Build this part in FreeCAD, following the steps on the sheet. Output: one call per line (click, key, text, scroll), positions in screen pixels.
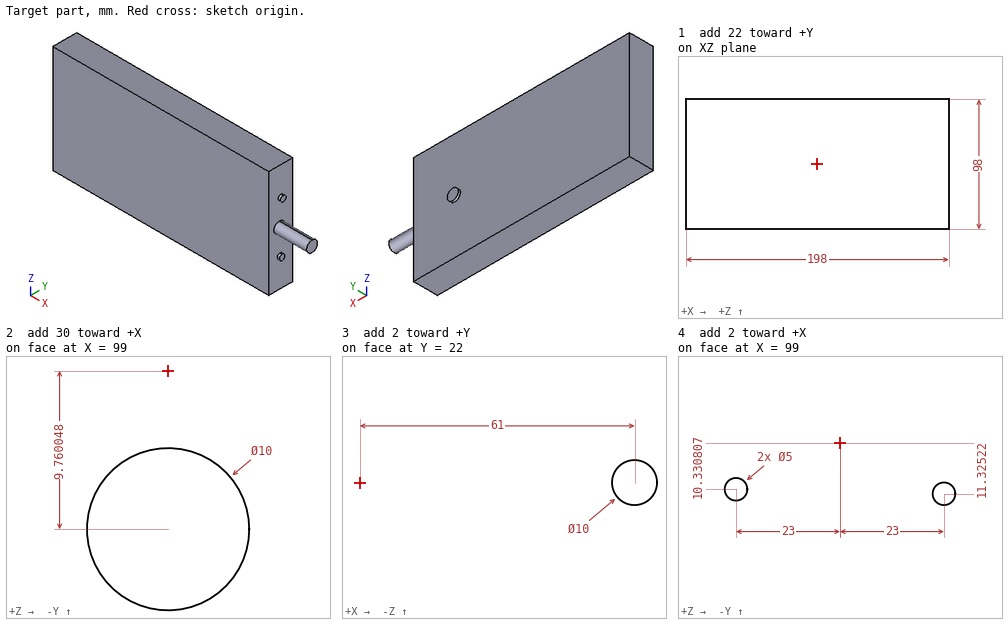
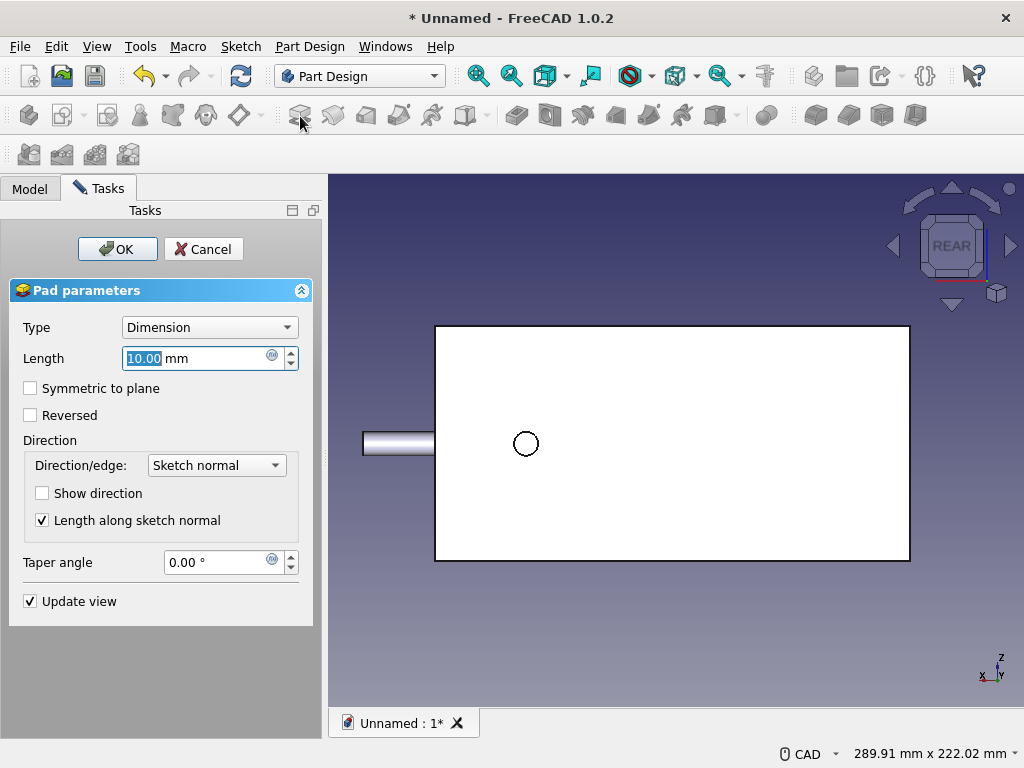
text(2)
key(Tab)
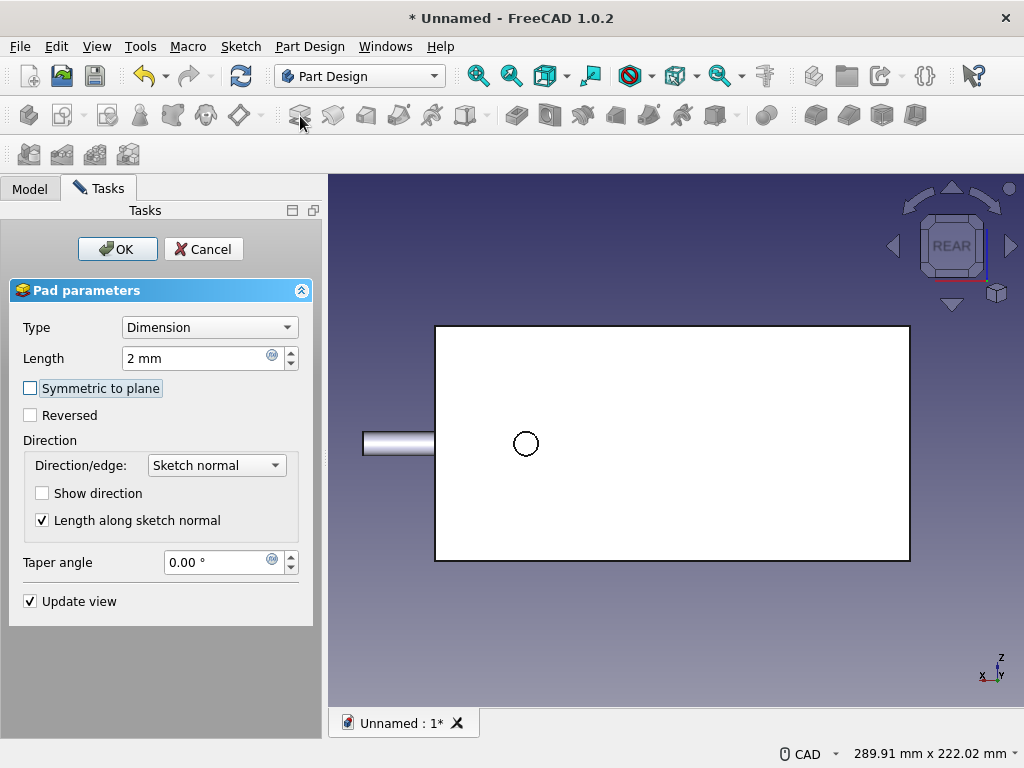
click(118, 249)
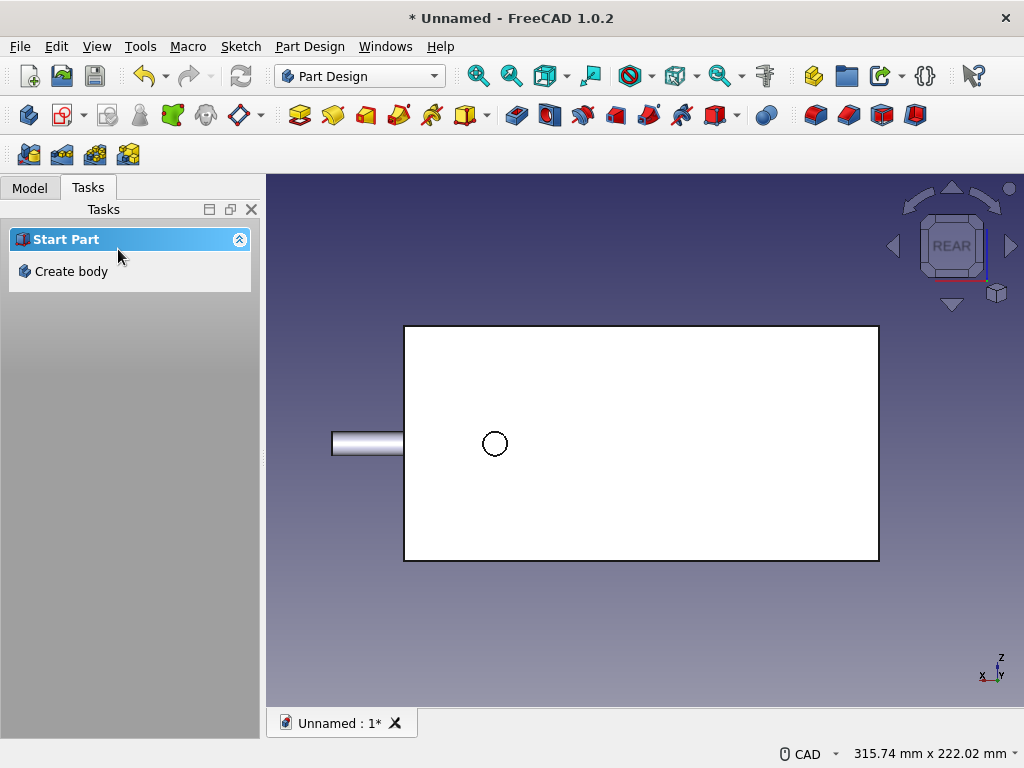
key(0)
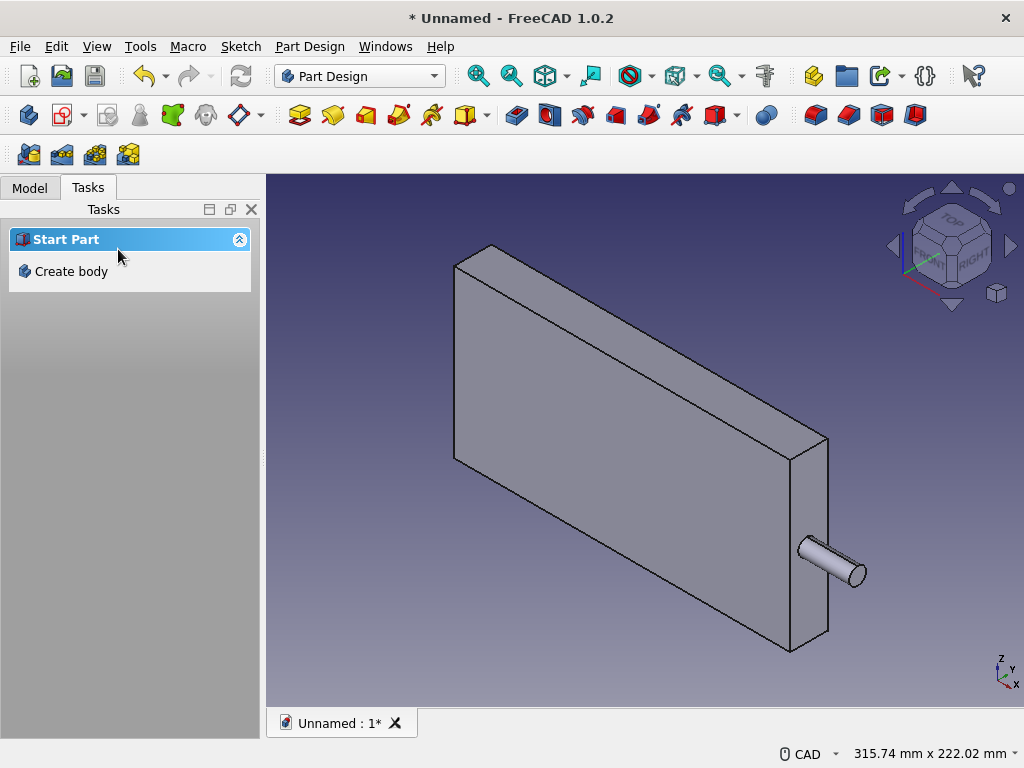
click(809, 490)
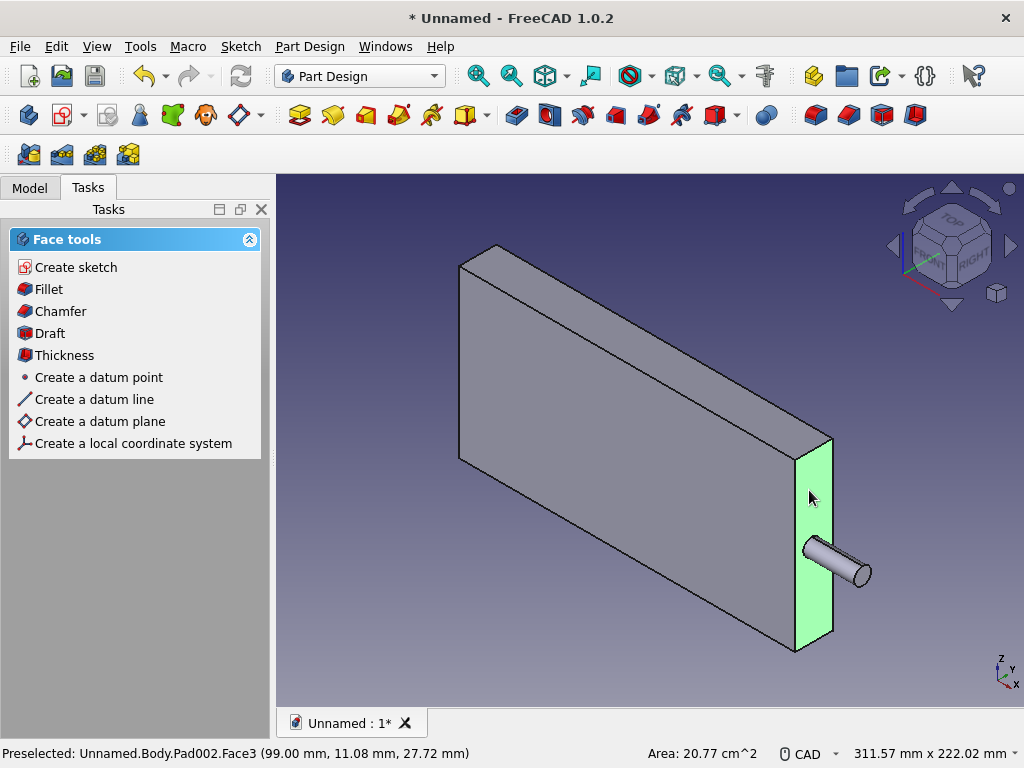
click(62, 116)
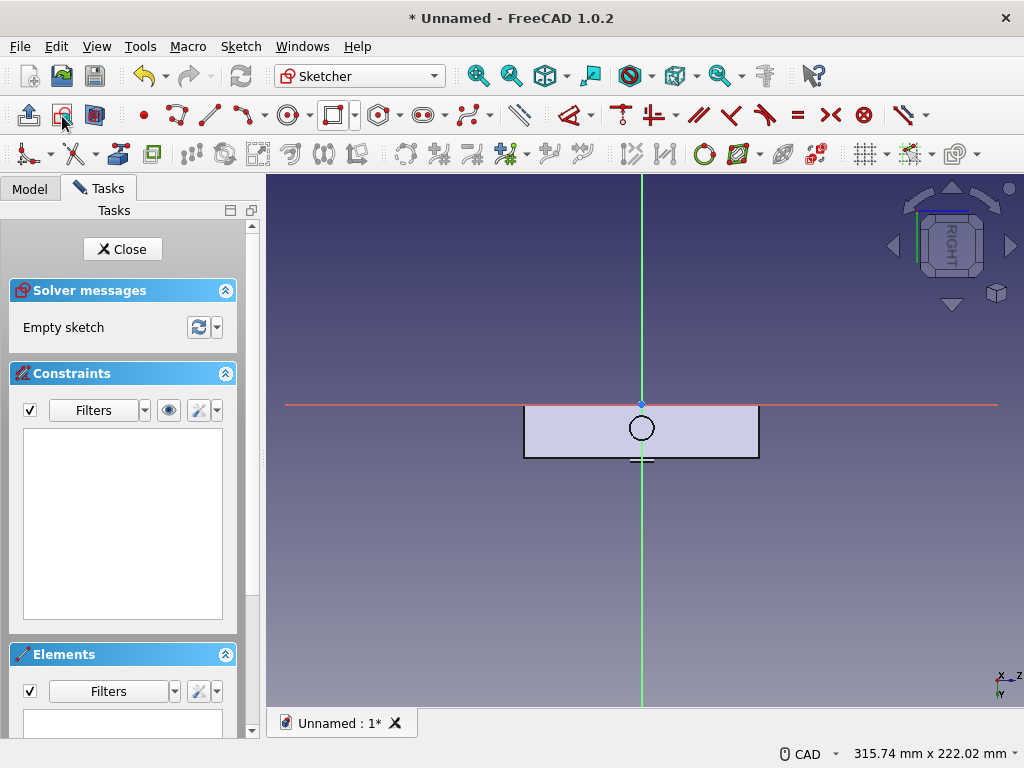
click(95, 116)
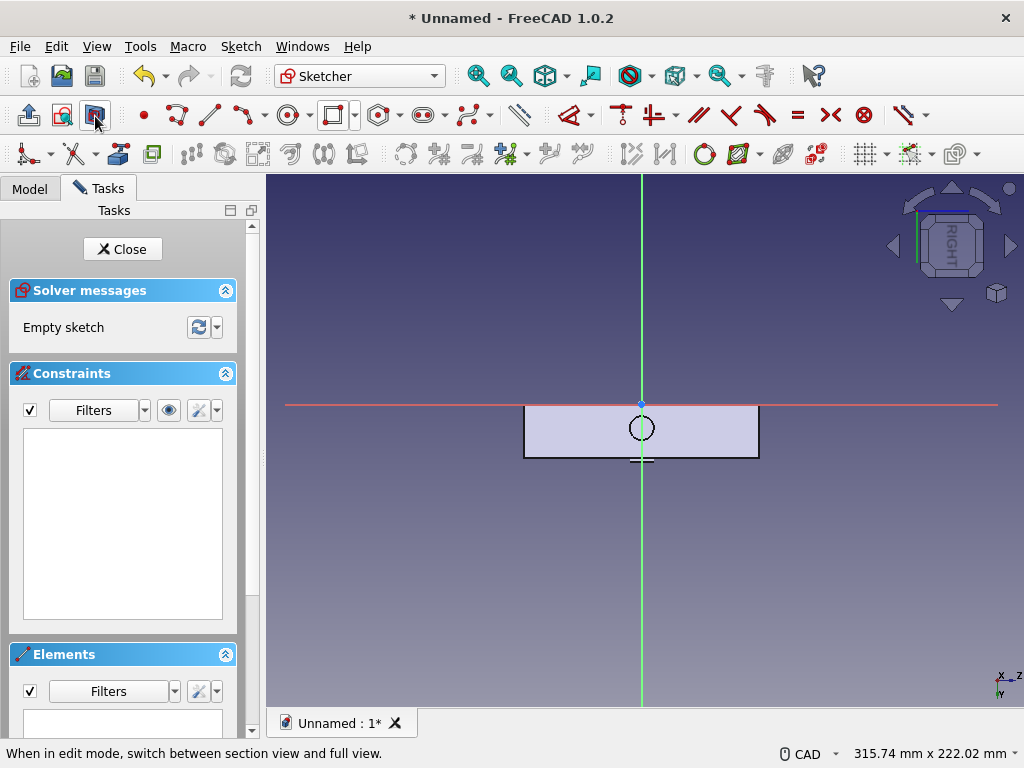
scroll(670, 413, up, 6)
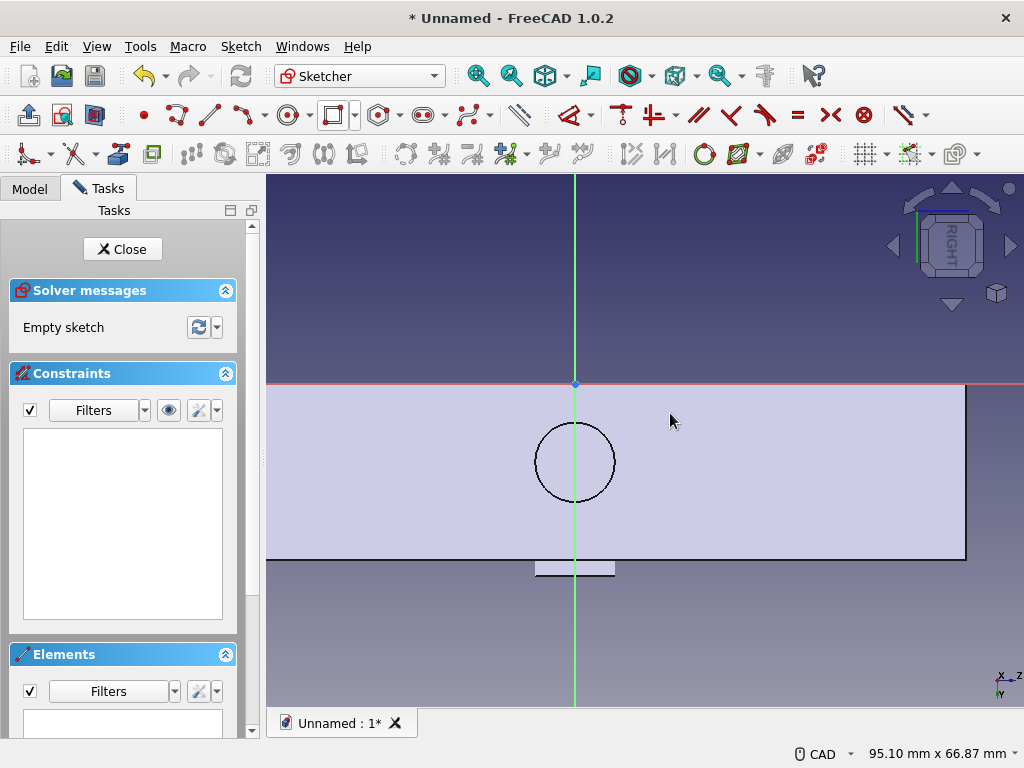
key(g)
key(c)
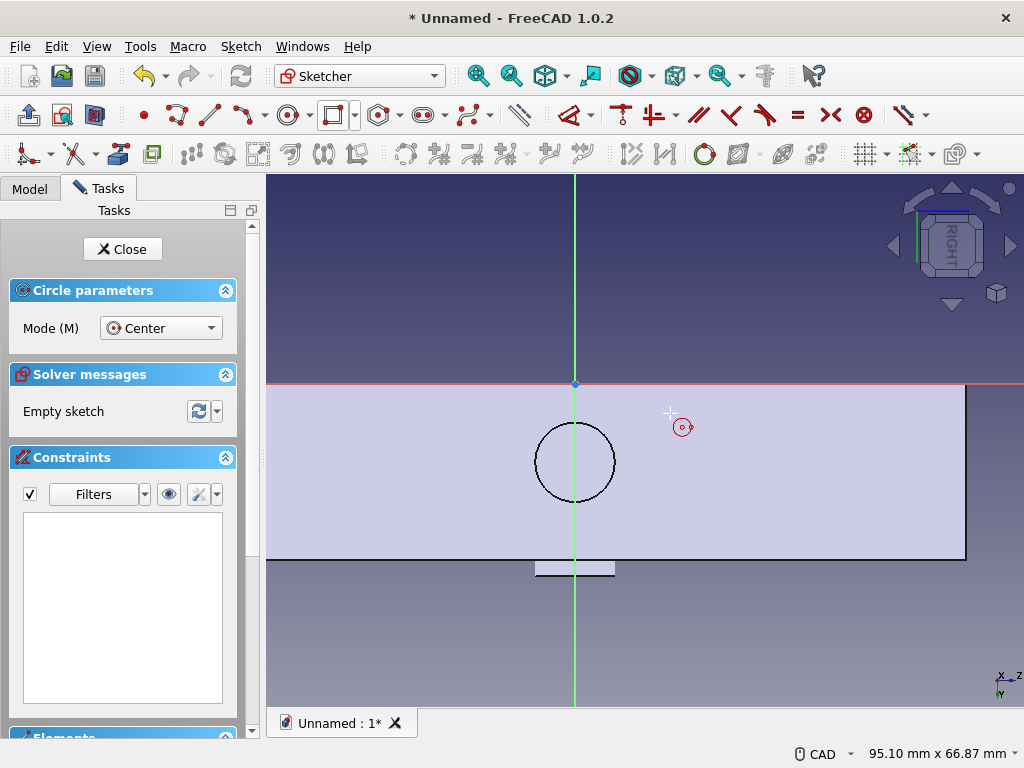
click(392, 467)
move(406, 453)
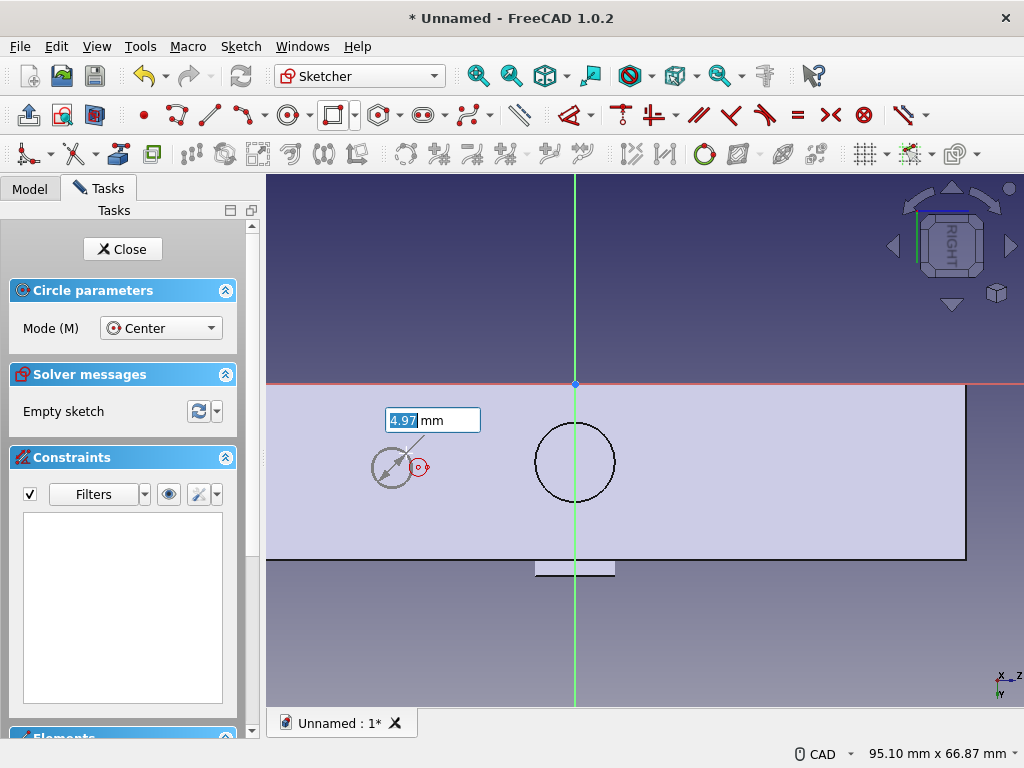
text(5)
key(Return)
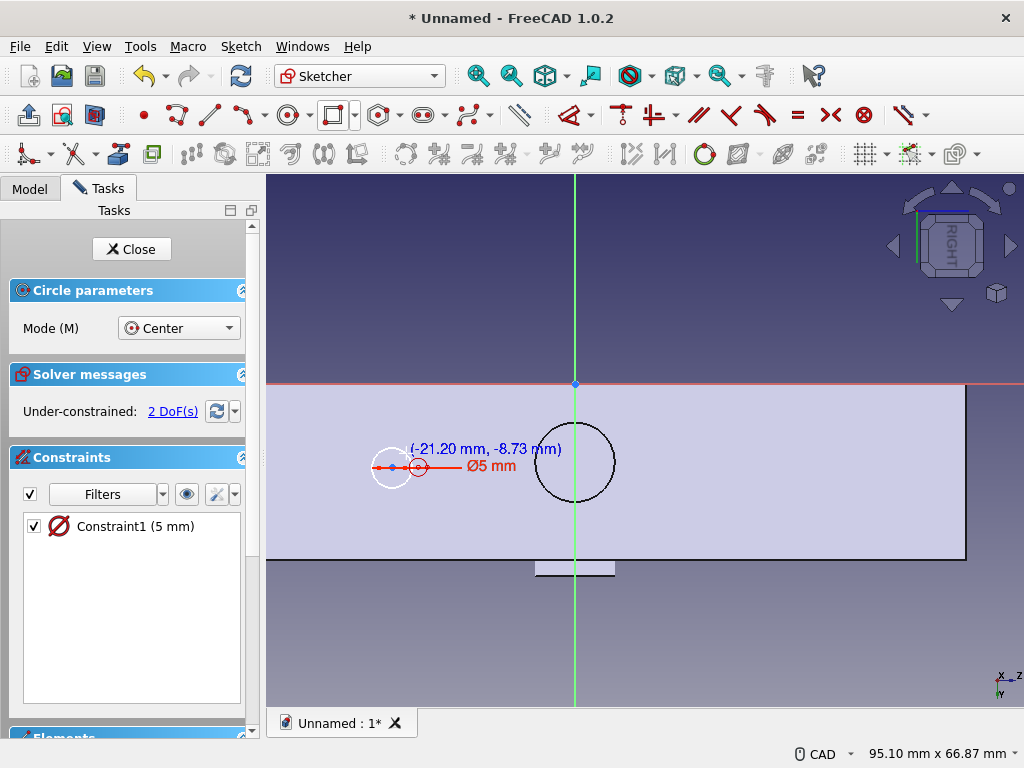
click(758, 475)
move(772, 461)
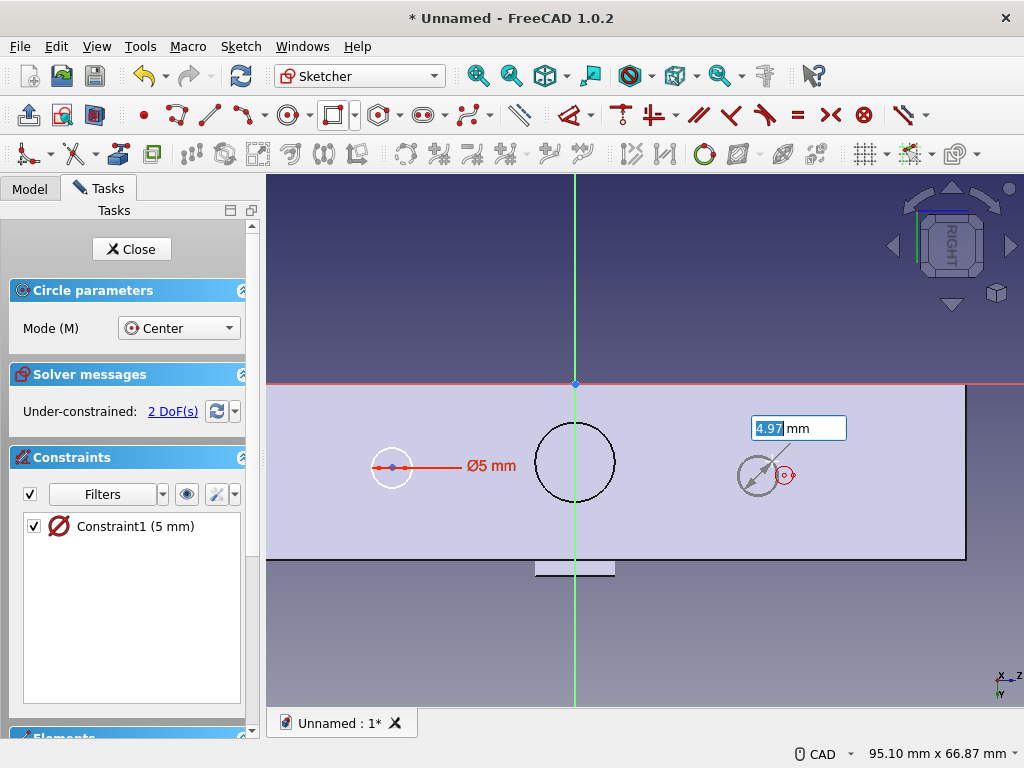
text(5)
key(Return)
key(Escape)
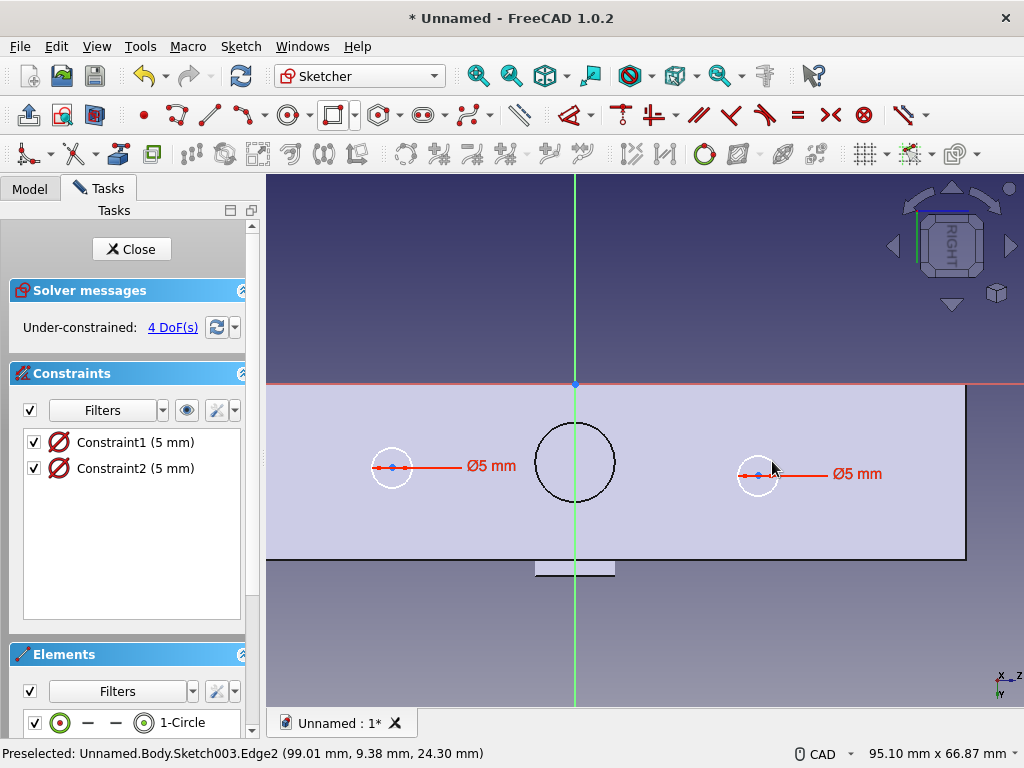
key(d)